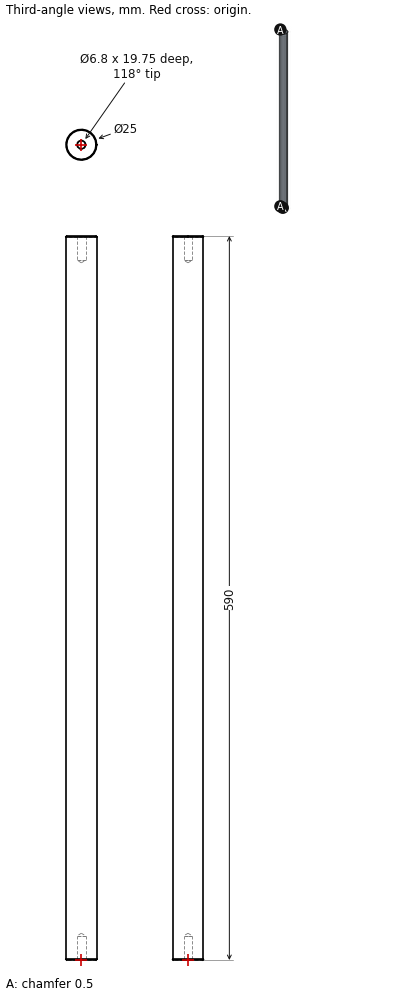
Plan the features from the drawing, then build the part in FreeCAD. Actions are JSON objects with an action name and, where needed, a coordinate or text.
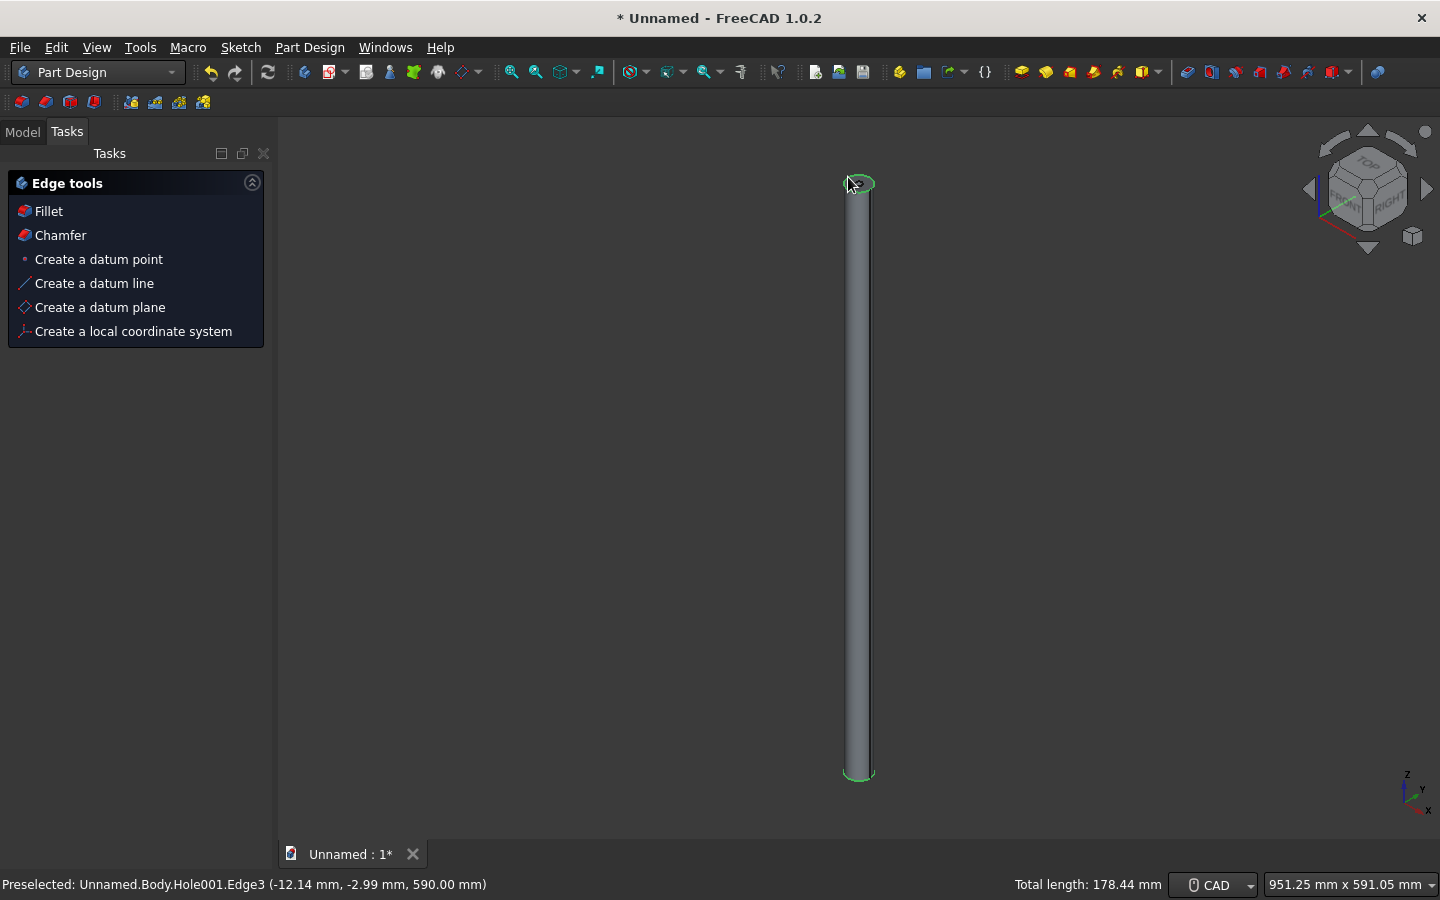
{"action": "left_click", "coordinate": [46, 102]}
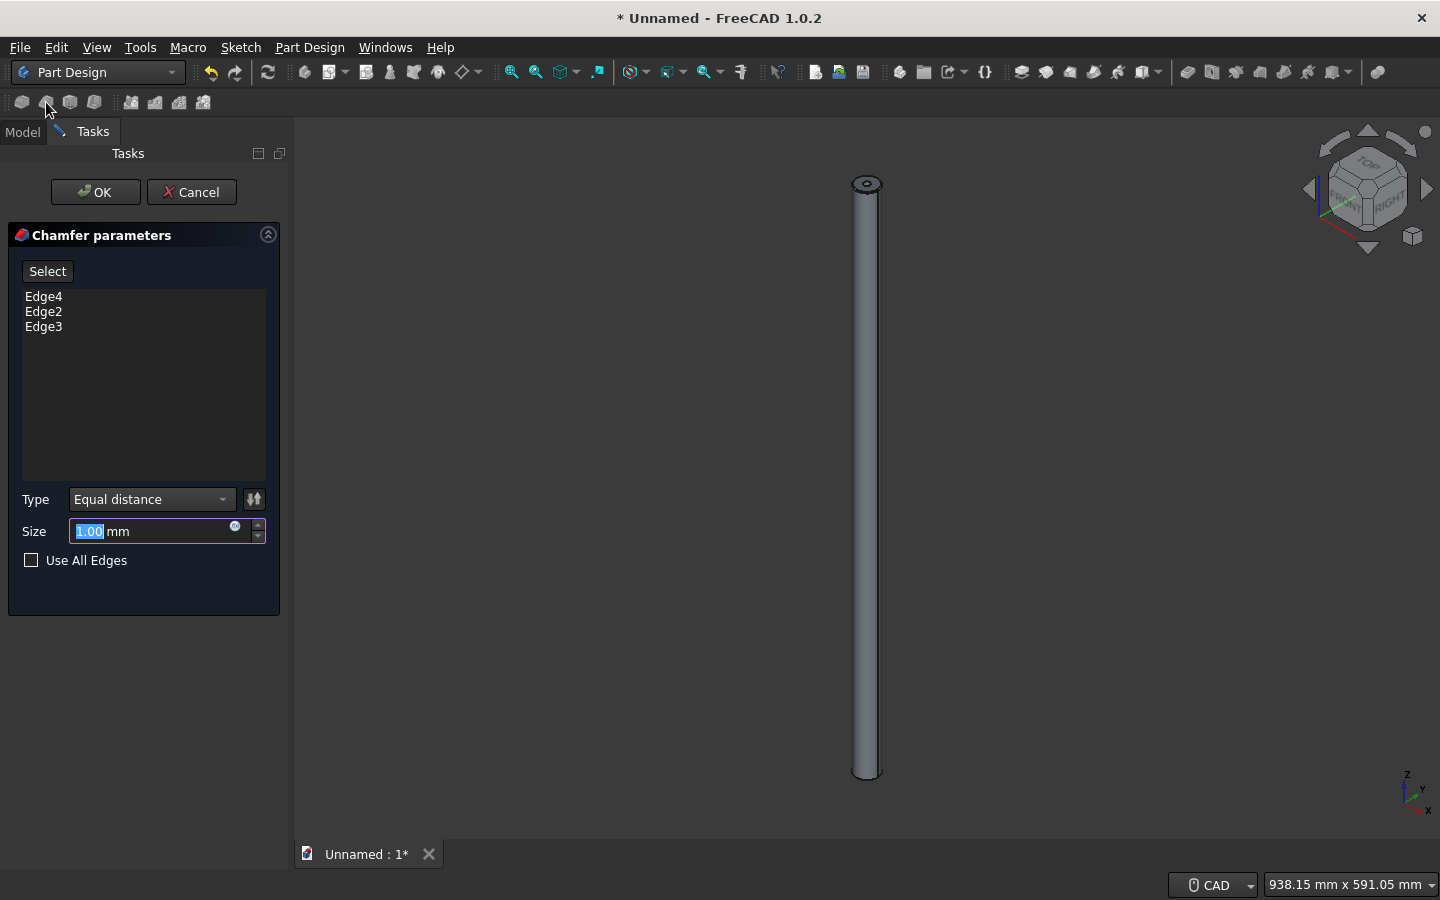
{"action": "type", "text": "0.5"}
{"action": "key", "text": "Tab"}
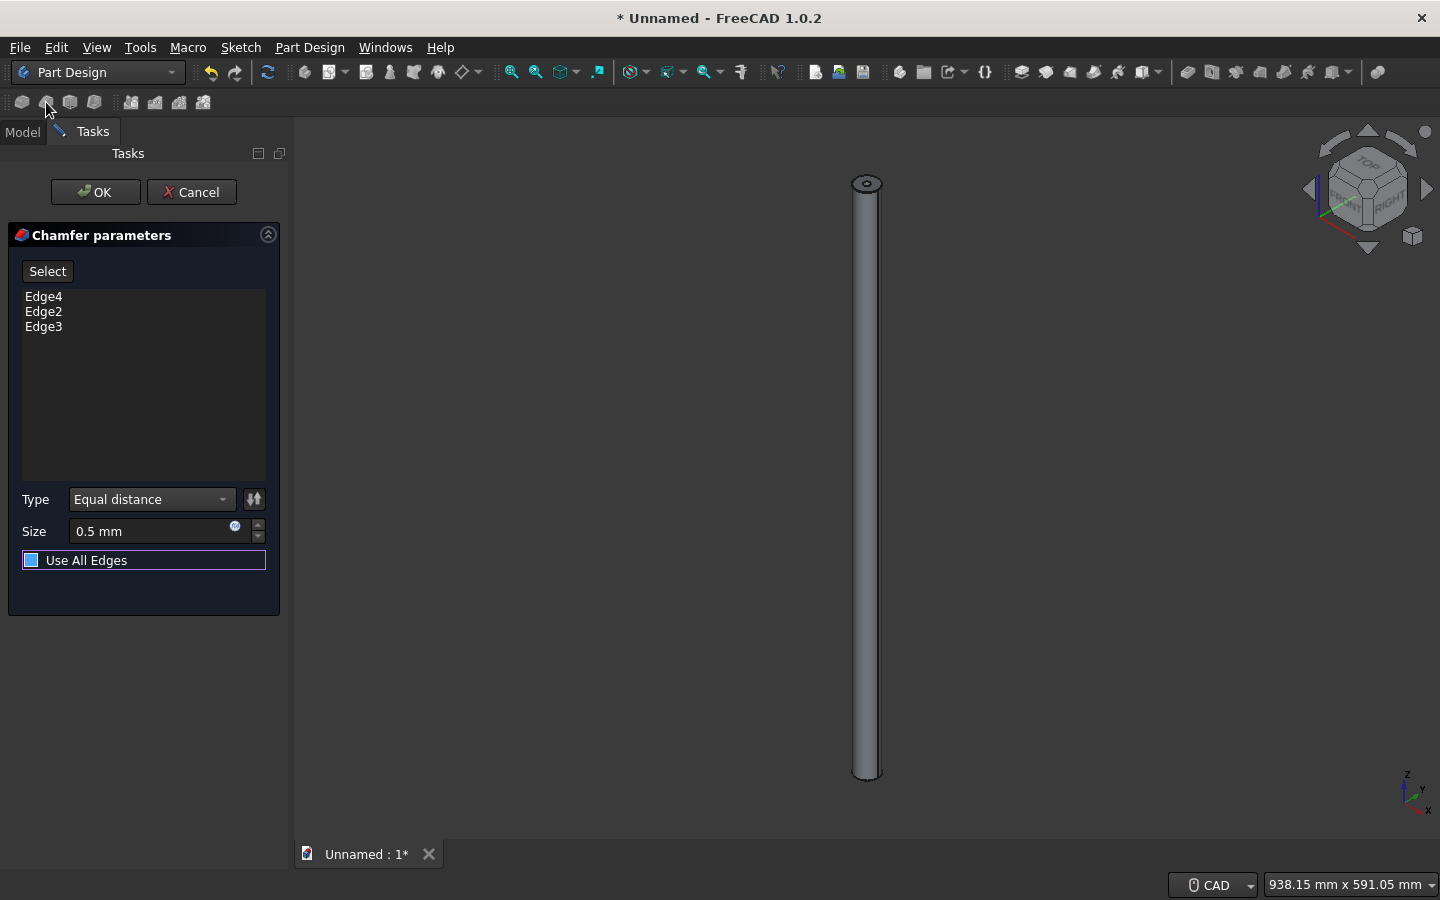
{"action": "left_click", "coordinate": [96, 192]}